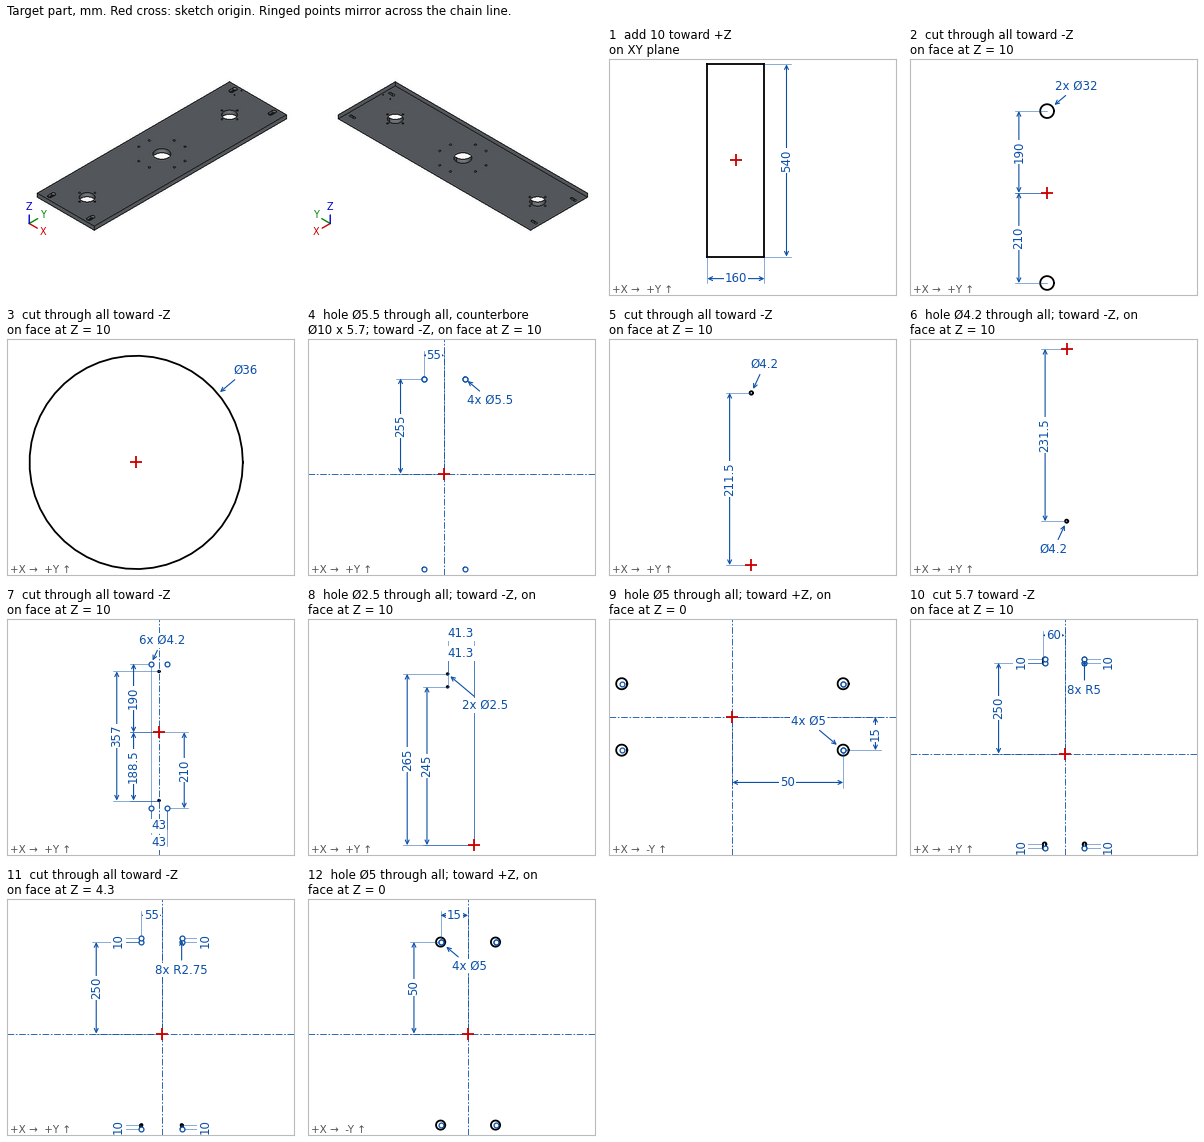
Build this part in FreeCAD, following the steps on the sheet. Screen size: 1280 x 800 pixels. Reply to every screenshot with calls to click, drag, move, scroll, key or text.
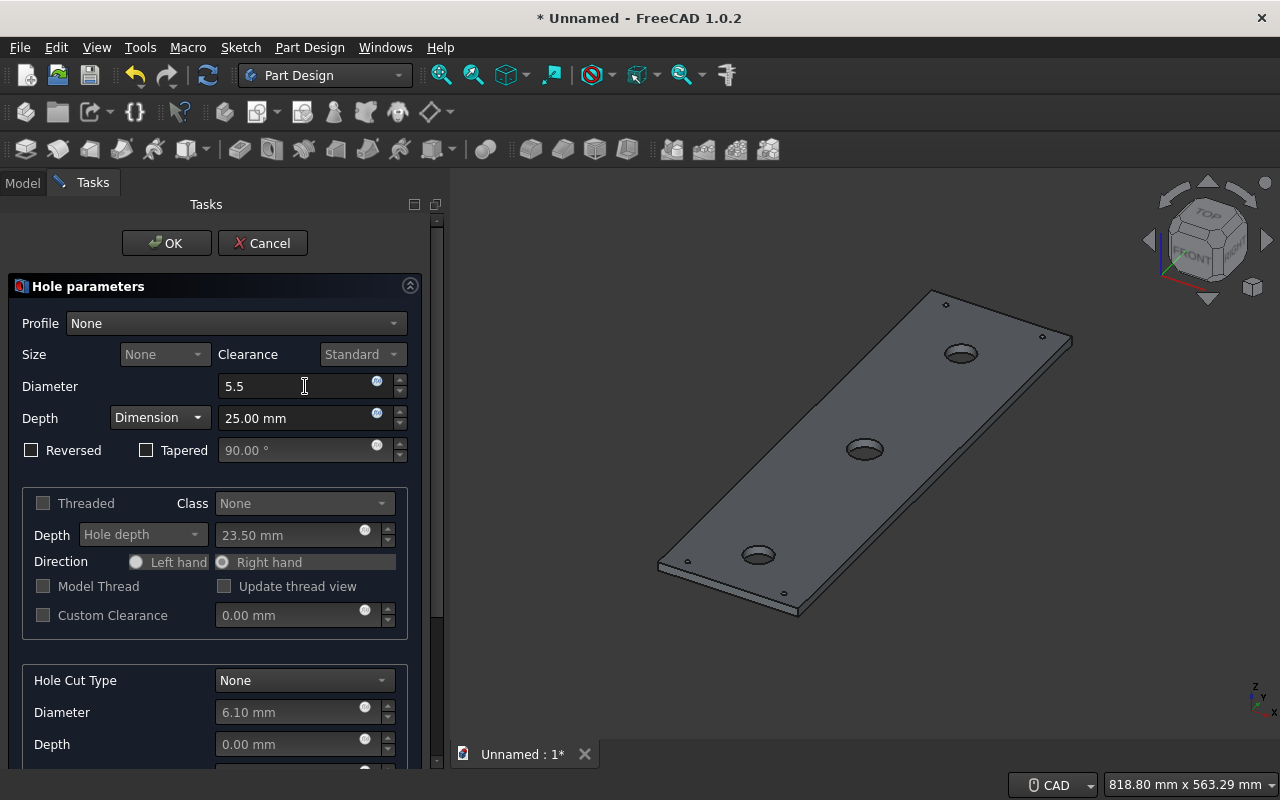
click(161, 418)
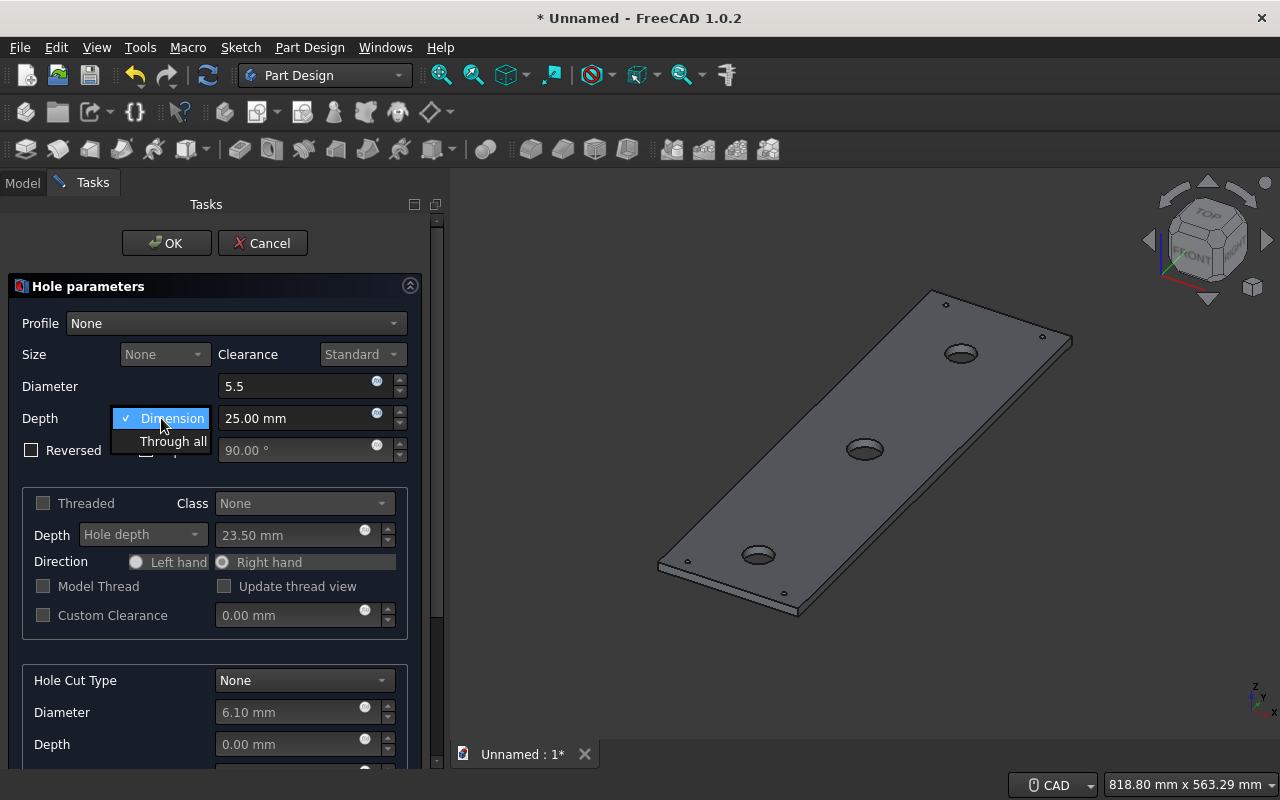
click(160, 442)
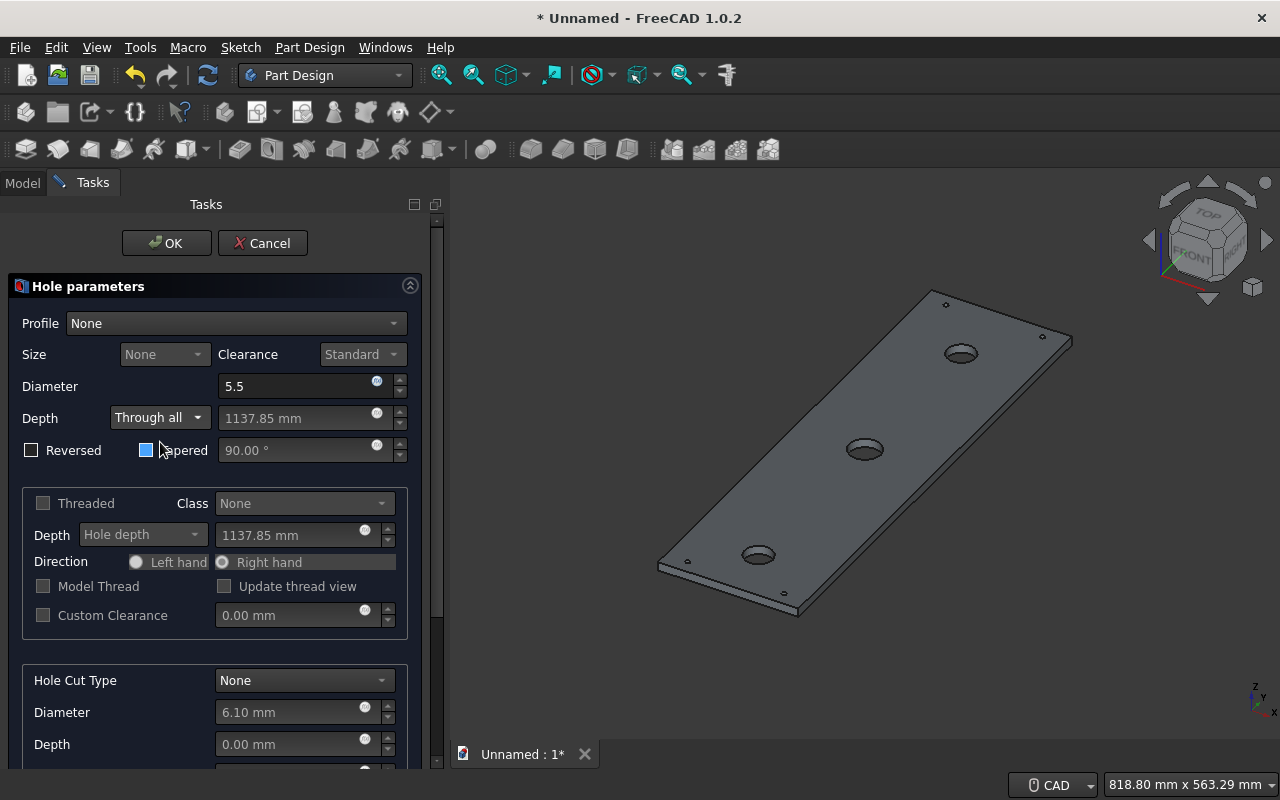
click(306, 680)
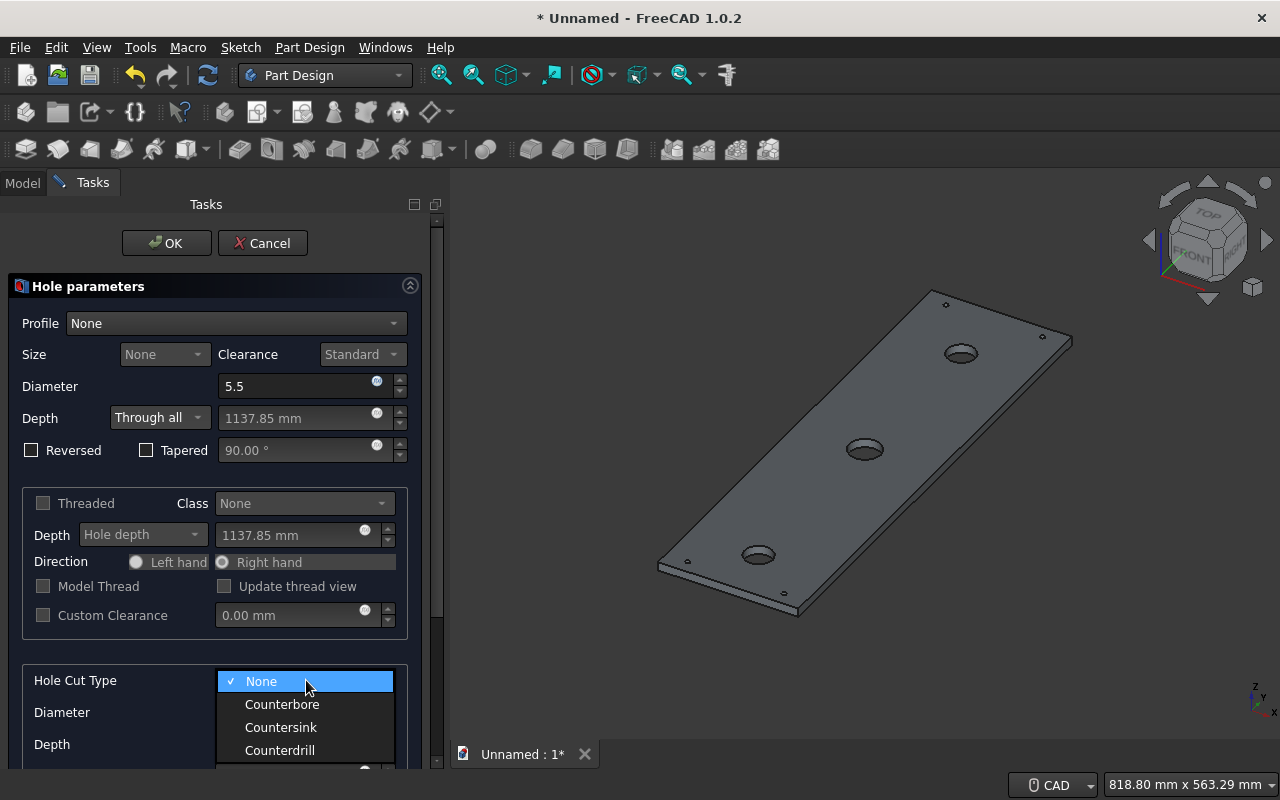
click(304, 704)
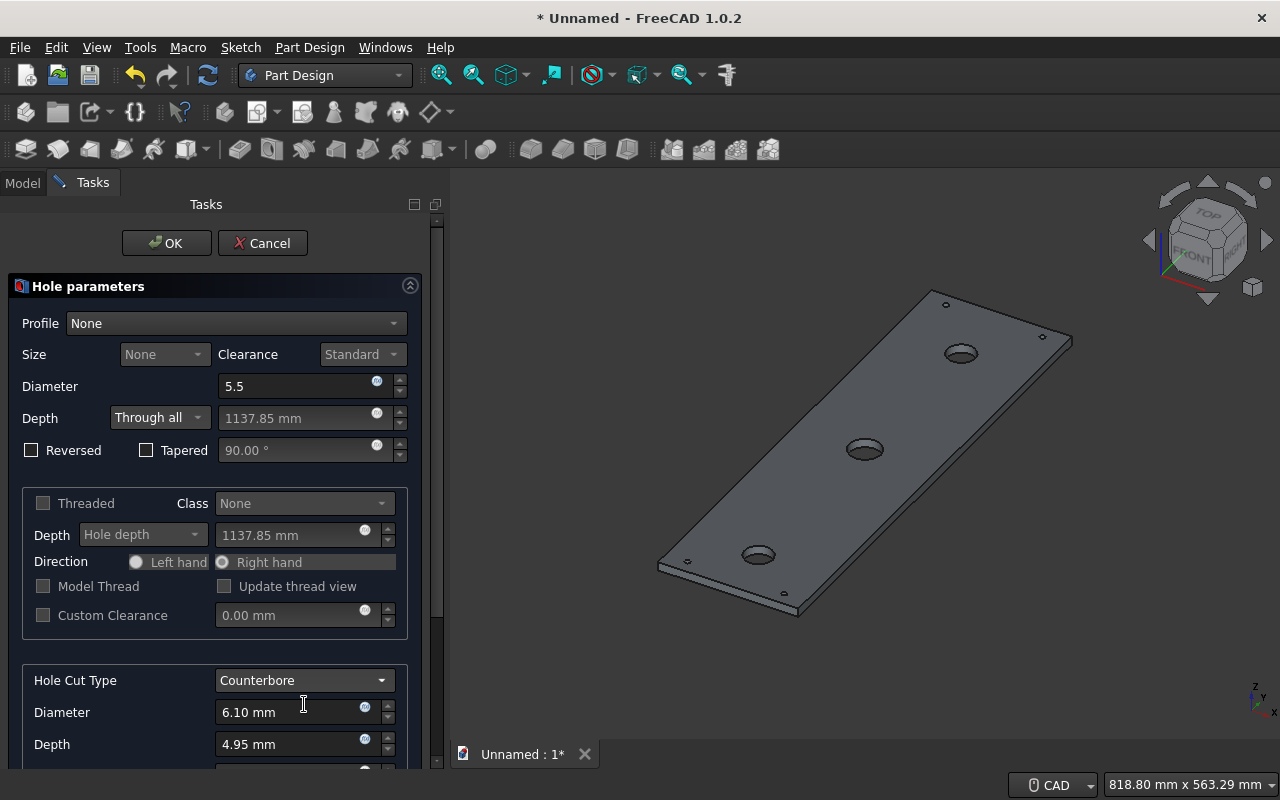
triple_click(298, 712)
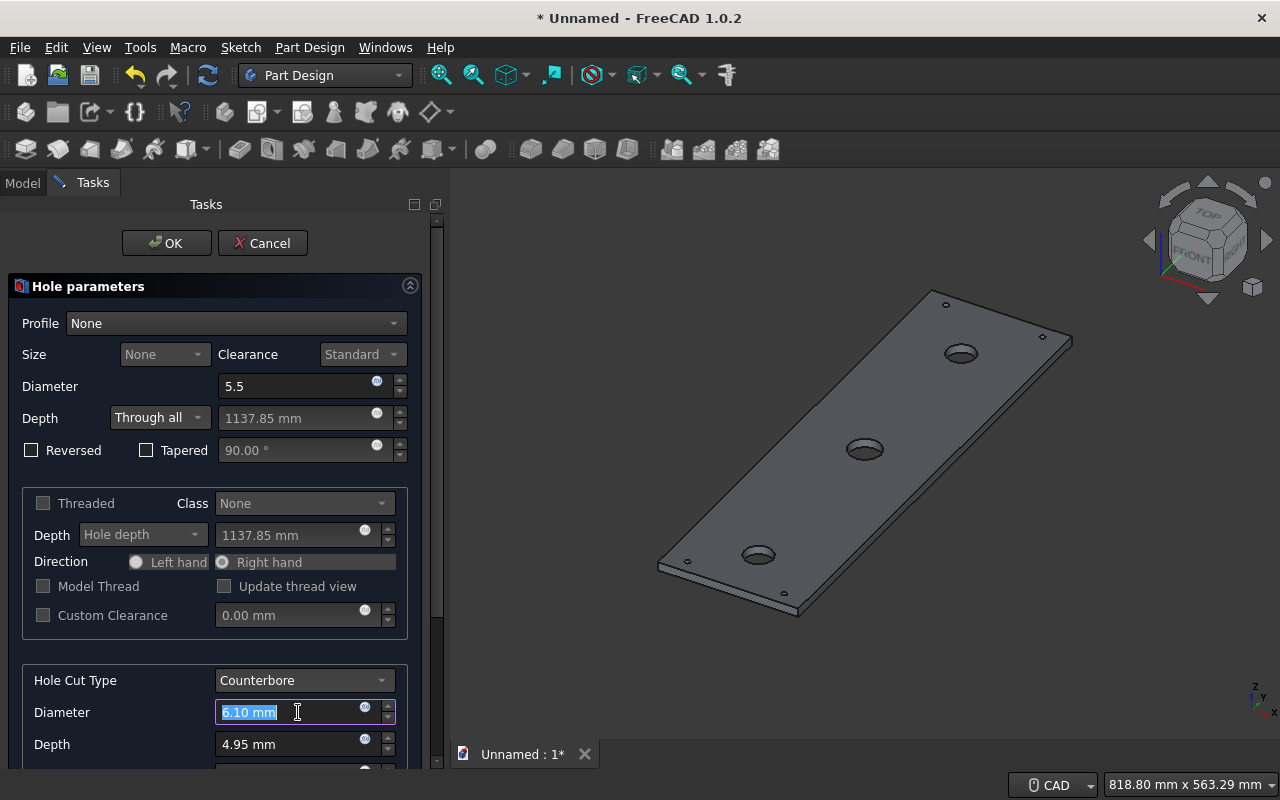
text(10)
key(Tab)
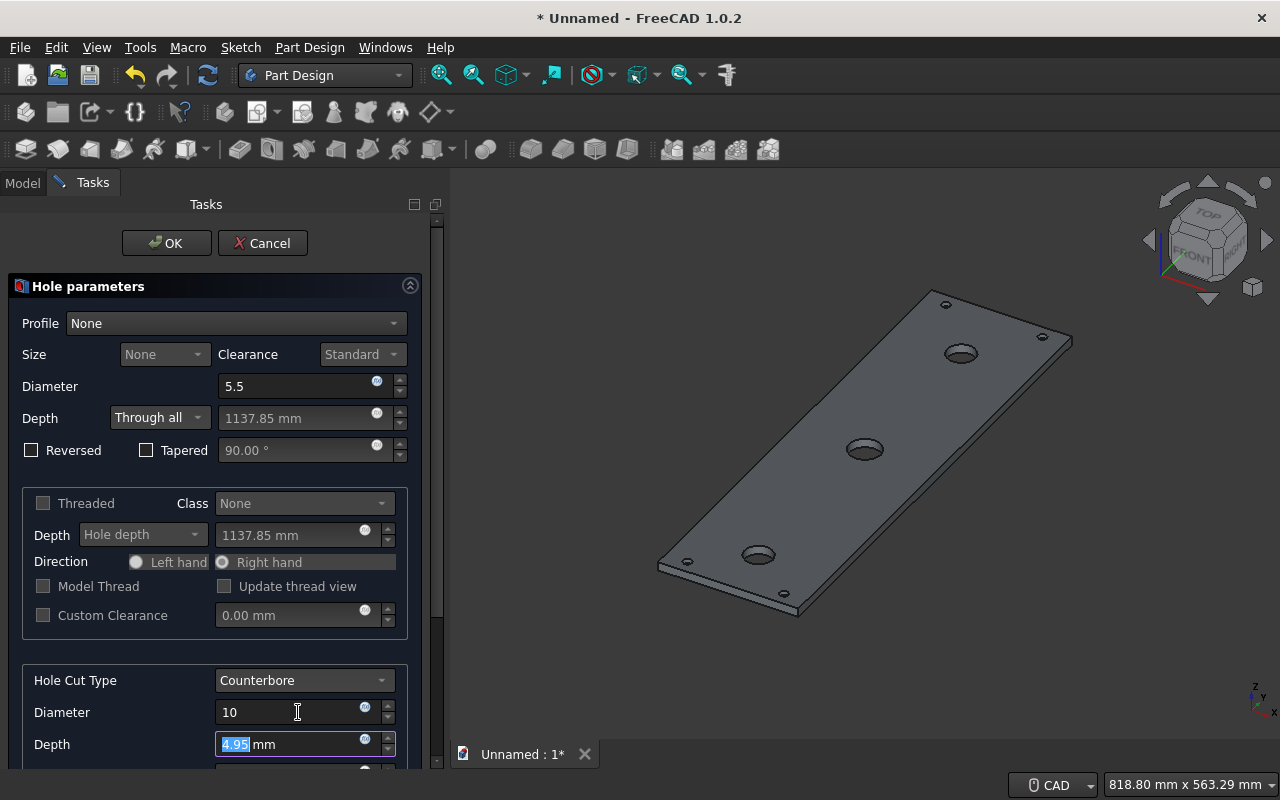
text(5.7)
key(Tab)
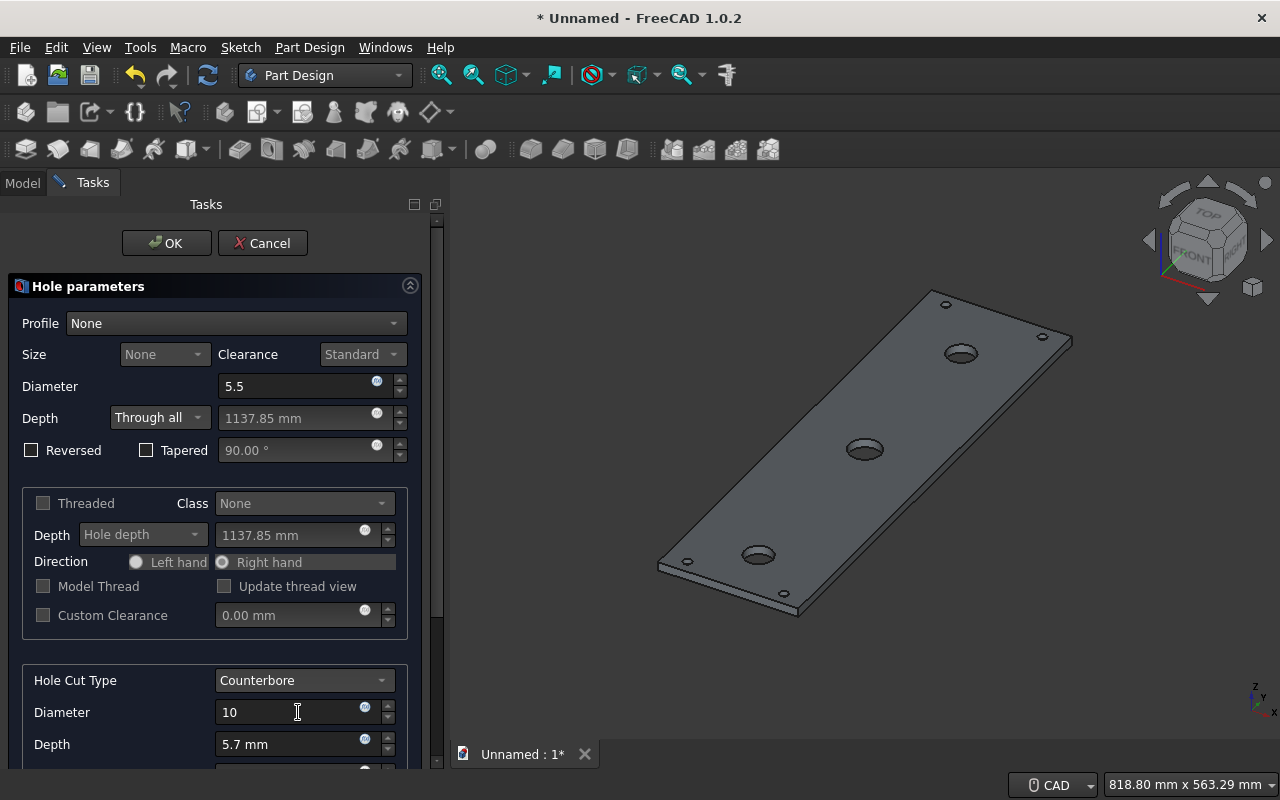
click(167, 243)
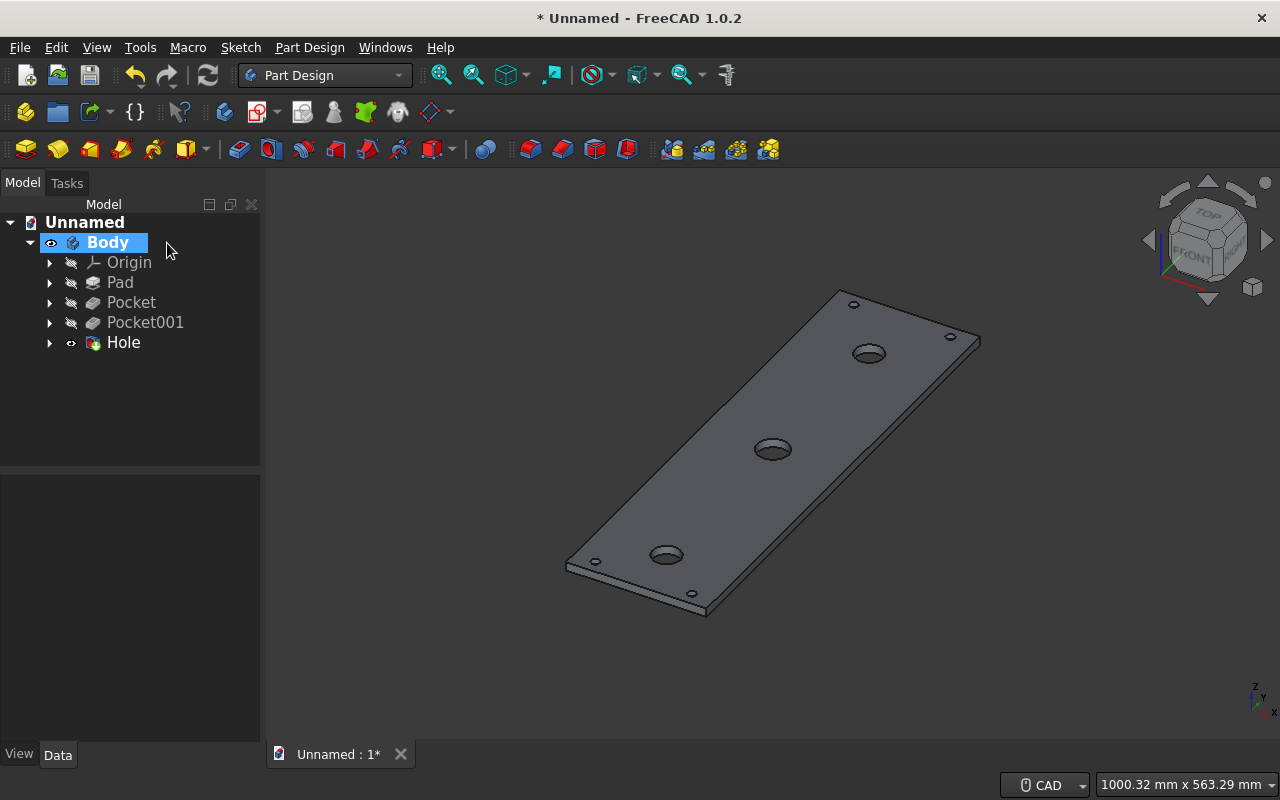
click(812, 410)